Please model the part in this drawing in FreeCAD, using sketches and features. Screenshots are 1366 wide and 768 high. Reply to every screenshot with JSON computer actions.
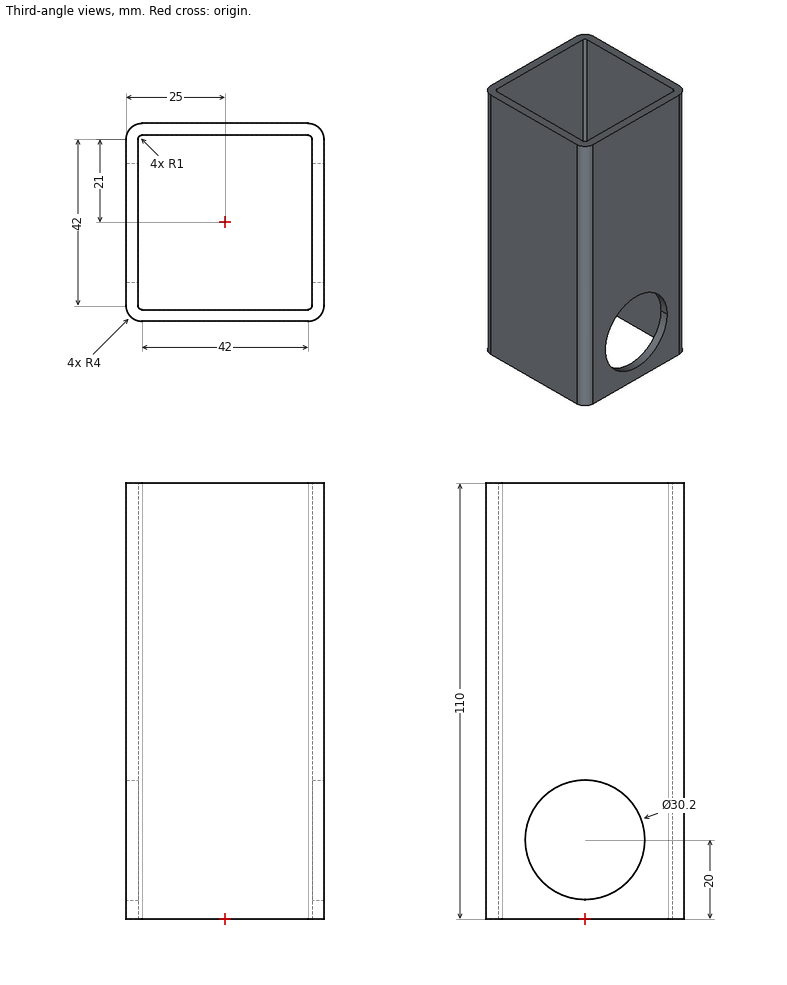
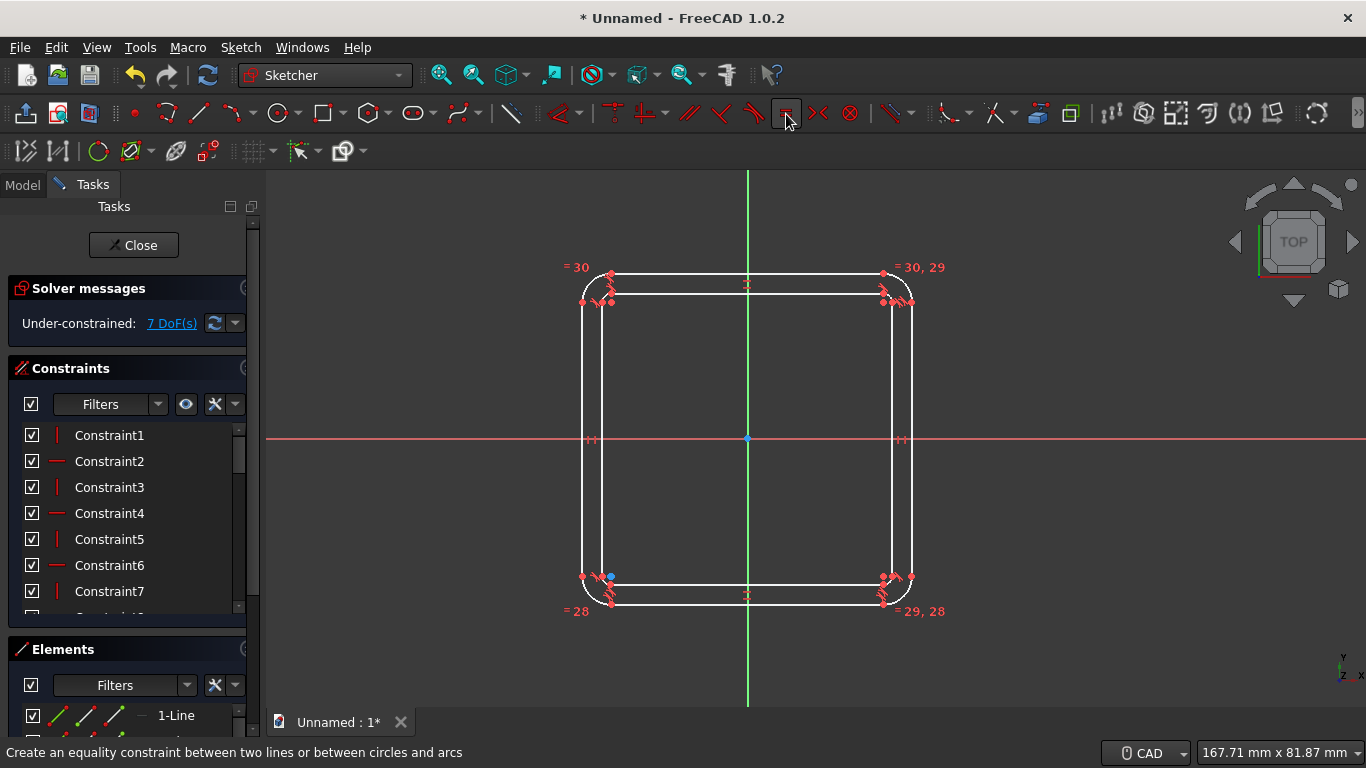
{"action": "scroll", "coordinate": [605, 296], "scroll_direction": "up", "scroll_amount": 4}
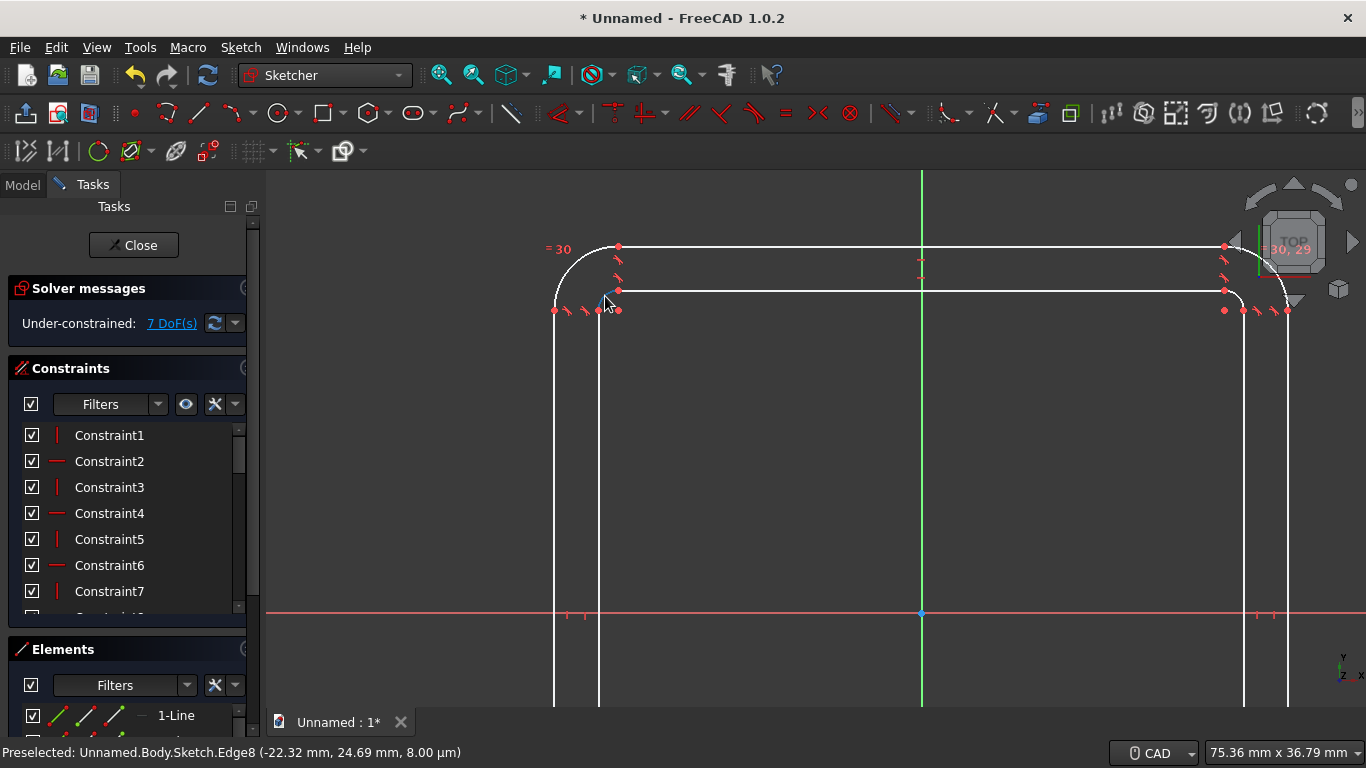
{"action": "left_click", "coordinate": [604, 296]}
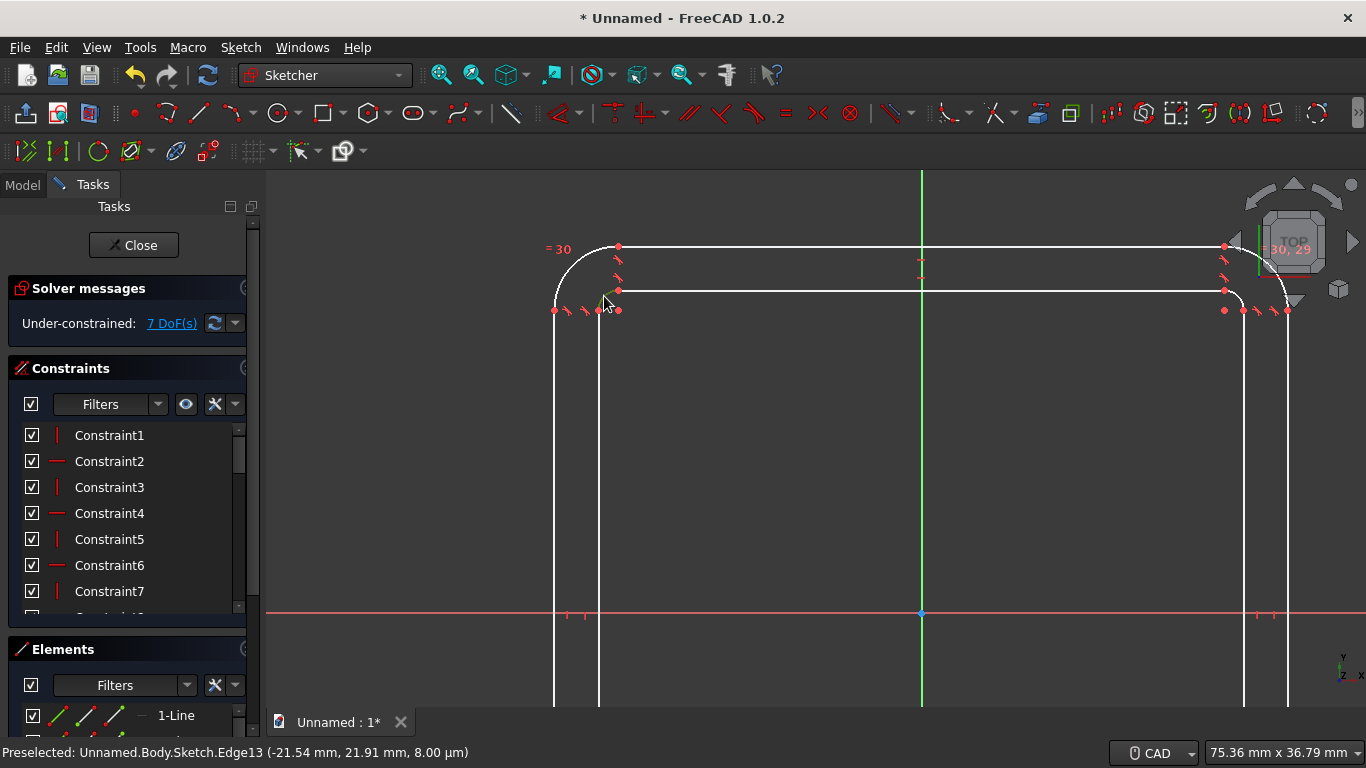
{"action": "scroll", "coordinate": [605, 296], "scroll_direction": "down", "scroll_amount": 4}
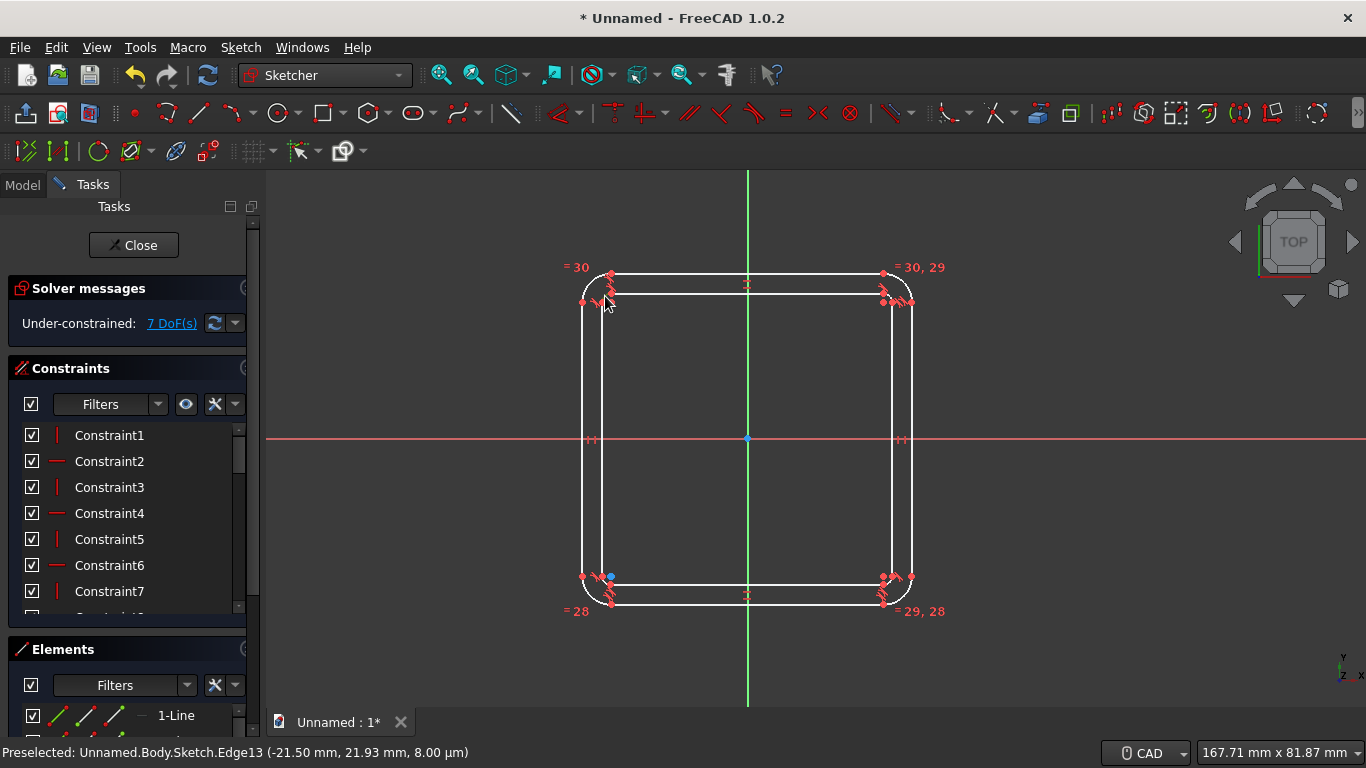
{"action": "scroll", "coordinate": [605, 582], "scroll_direction": "up", "scroll_amount": 4}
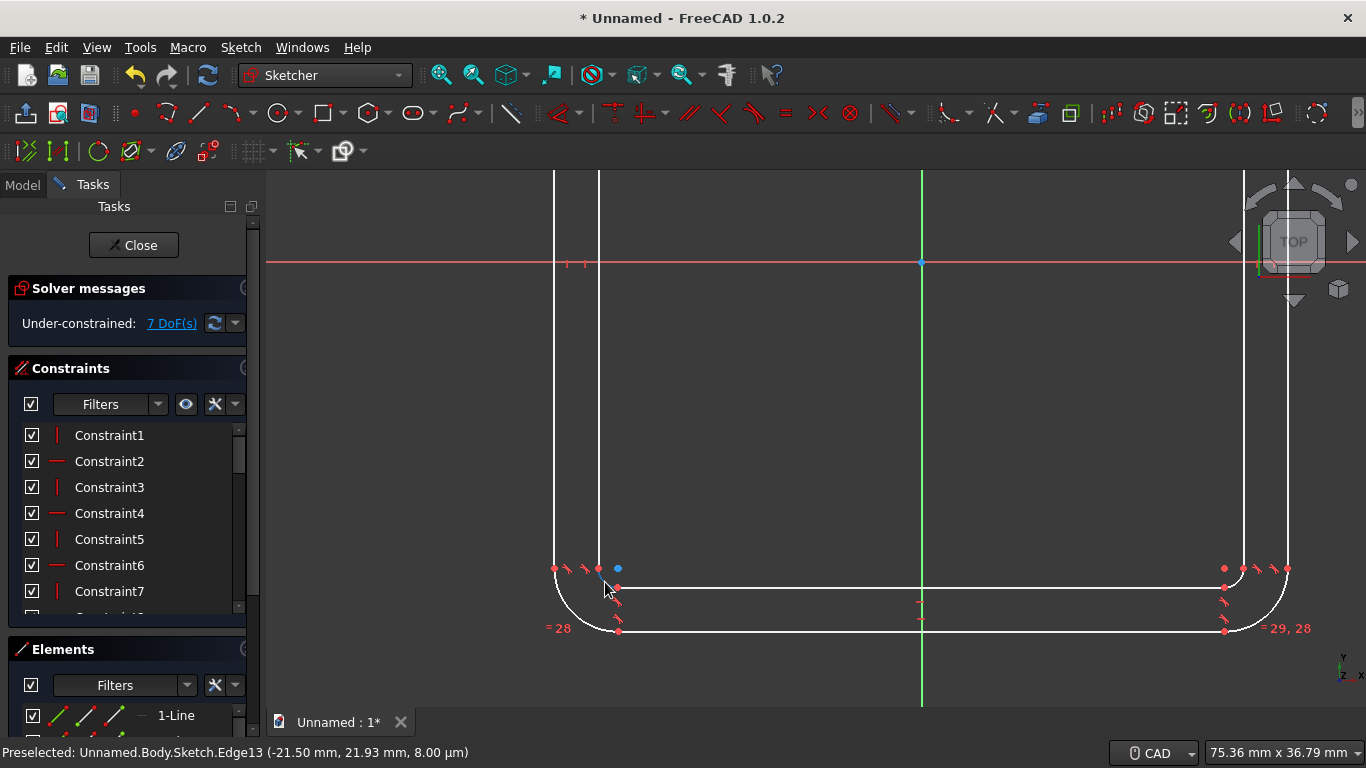
{"action": "left_click", "coordinate": [604, 582]}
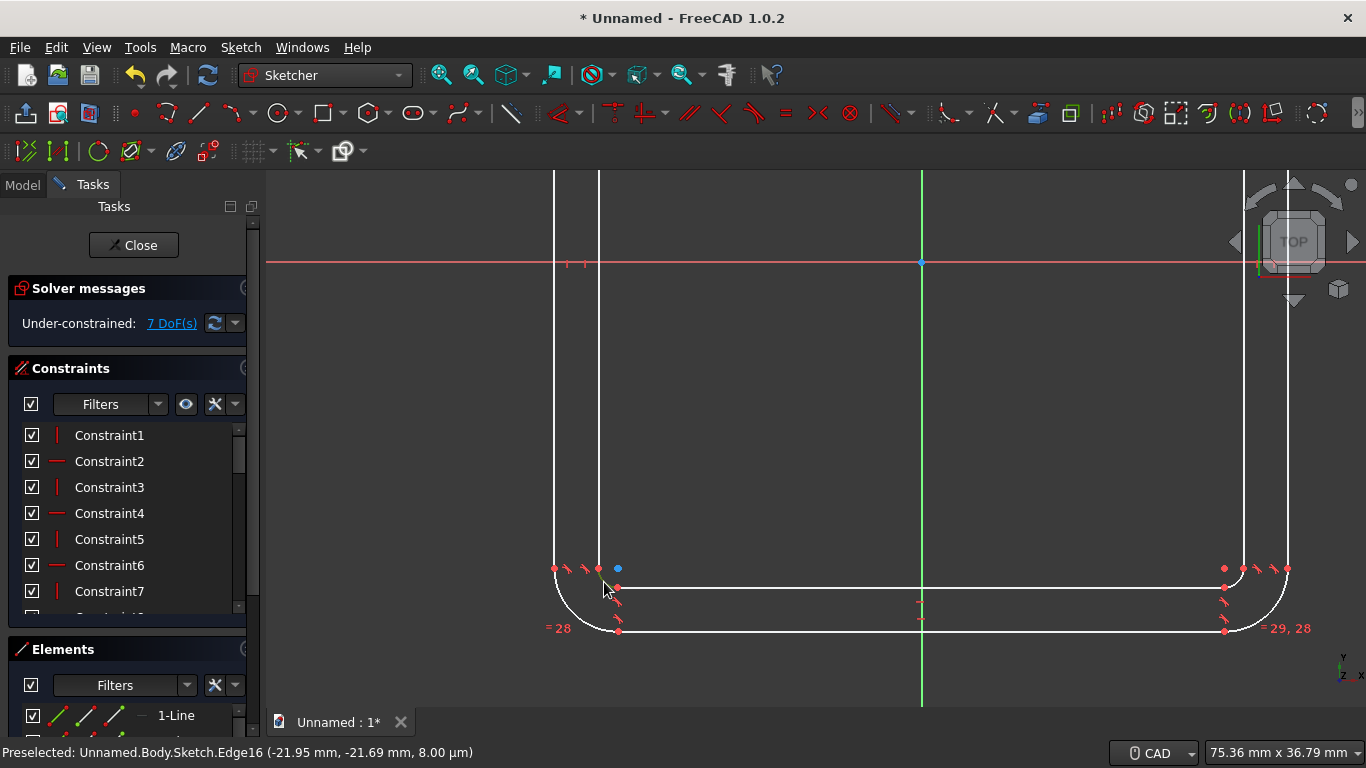
{"action": "left_click", "coordinate": [786, 114]}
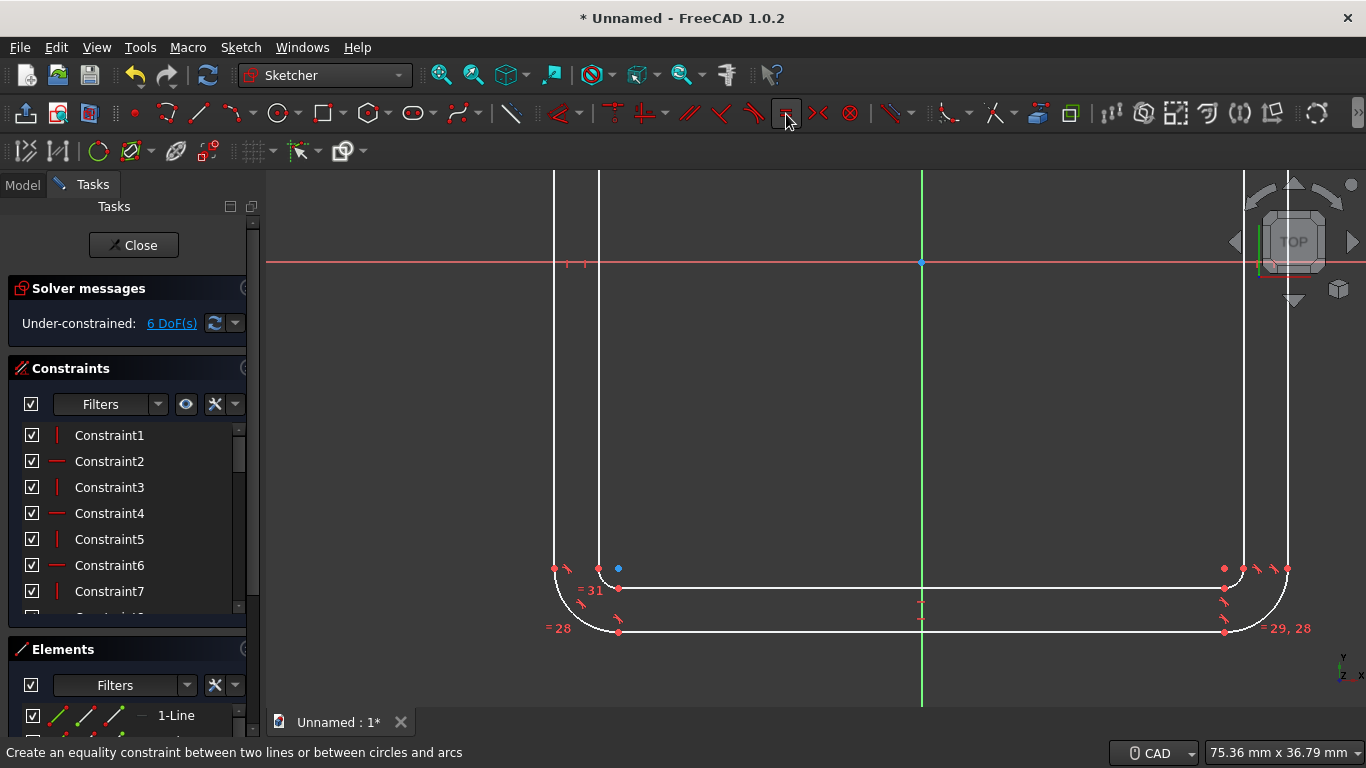
{"action": "left_click", "coordinate": [558, 114]}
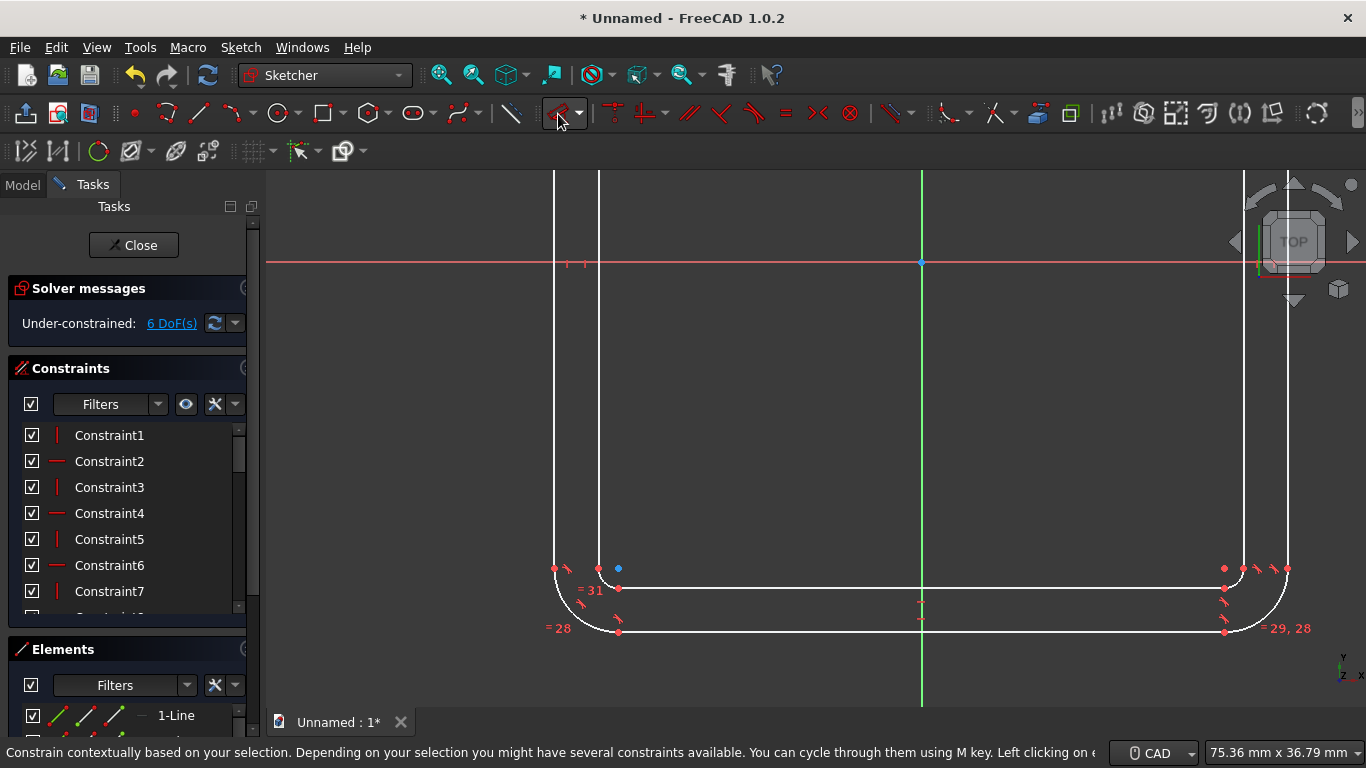
{"action": "left_click", "coordinate": [561, 597]}
{"action": "left_click", "coordinate": [532, 611]}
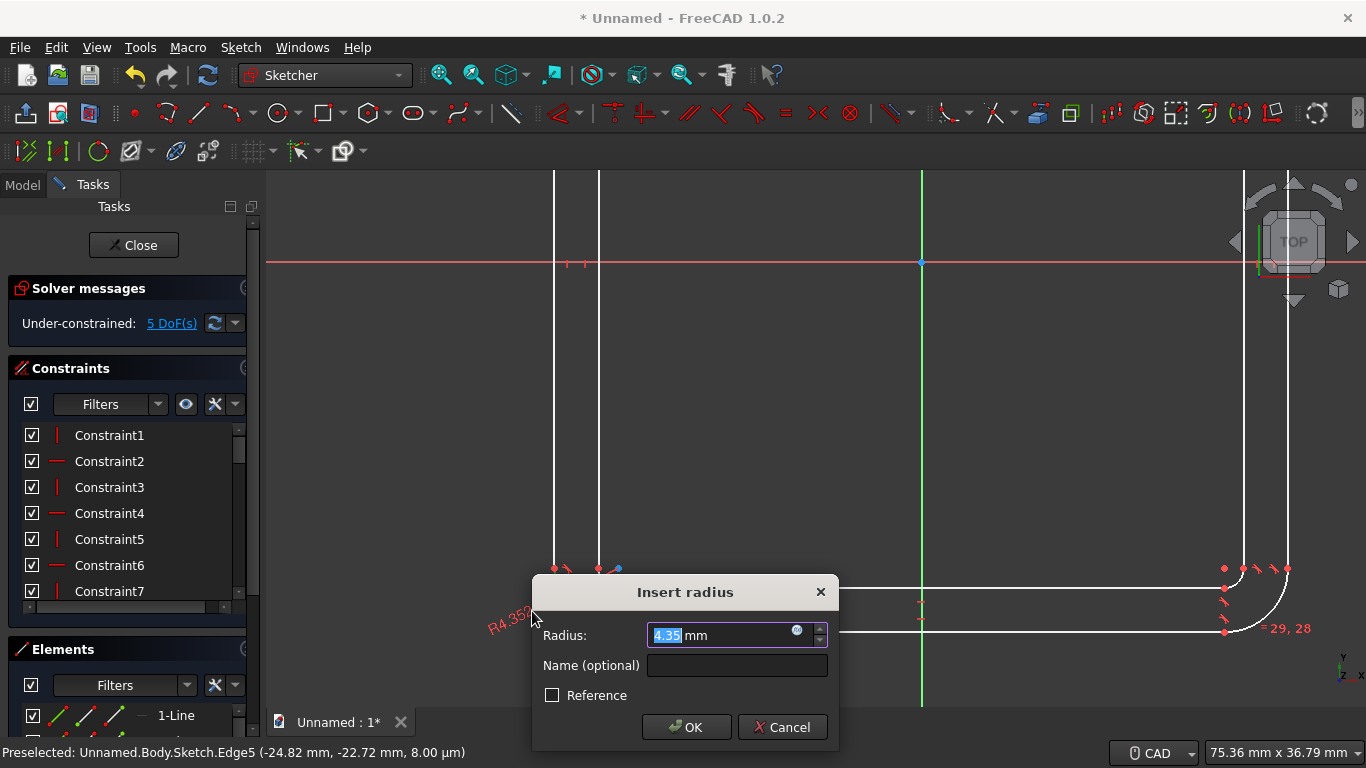
{"action": "type", "text": "4"}
{"action": "key", "text": "Return"}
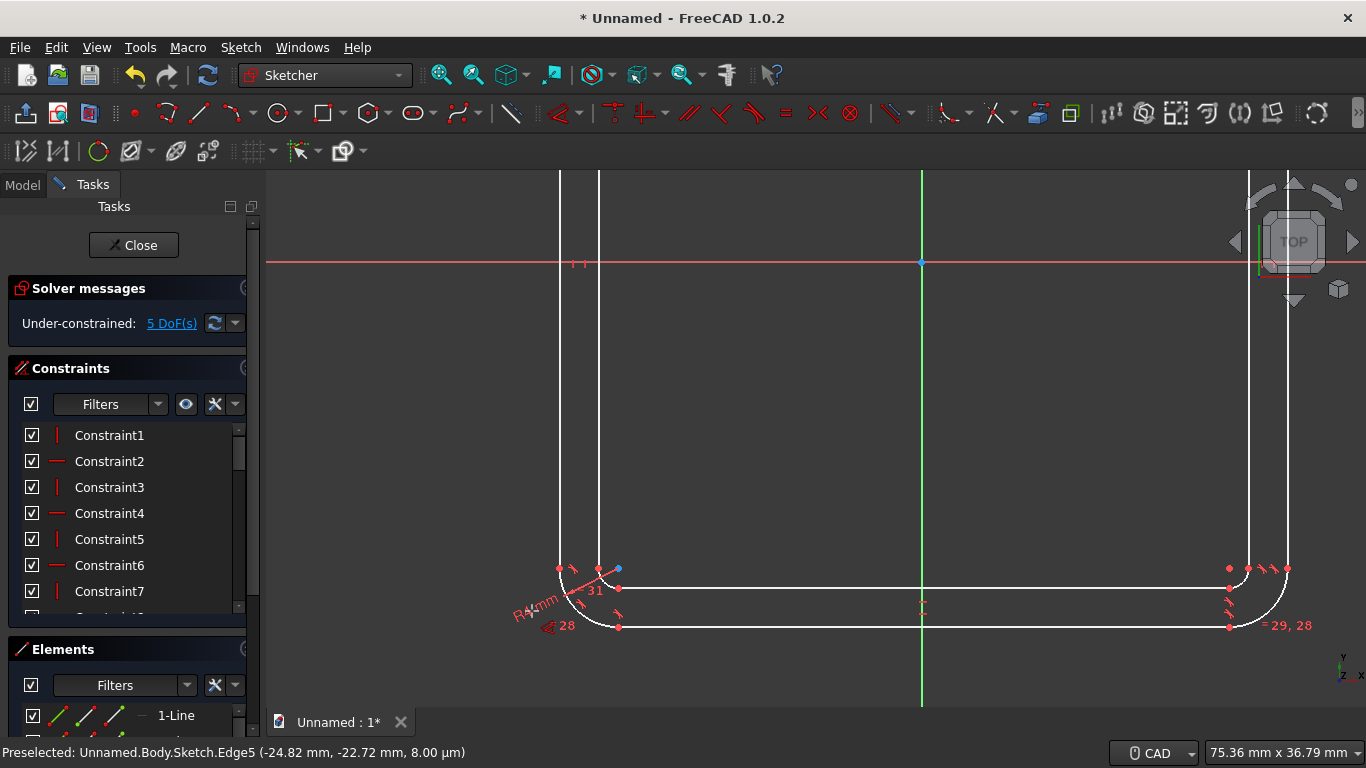
{"action": "scroll", "coordinate": [605, 582], "scroll_direction": "down", "scroll_amount": 4}